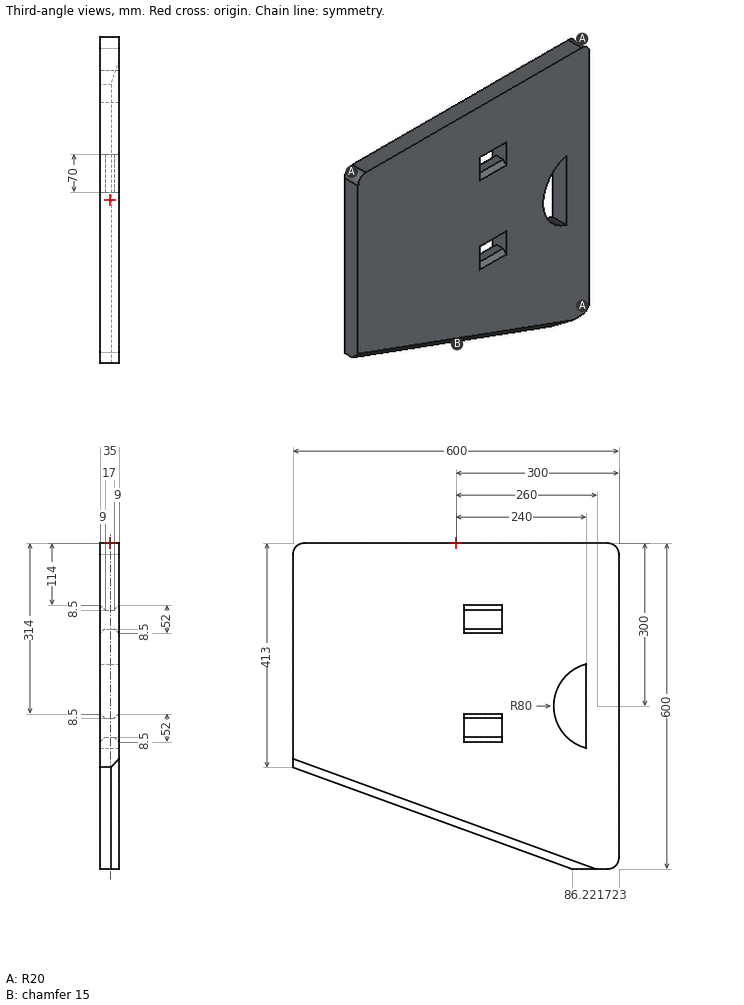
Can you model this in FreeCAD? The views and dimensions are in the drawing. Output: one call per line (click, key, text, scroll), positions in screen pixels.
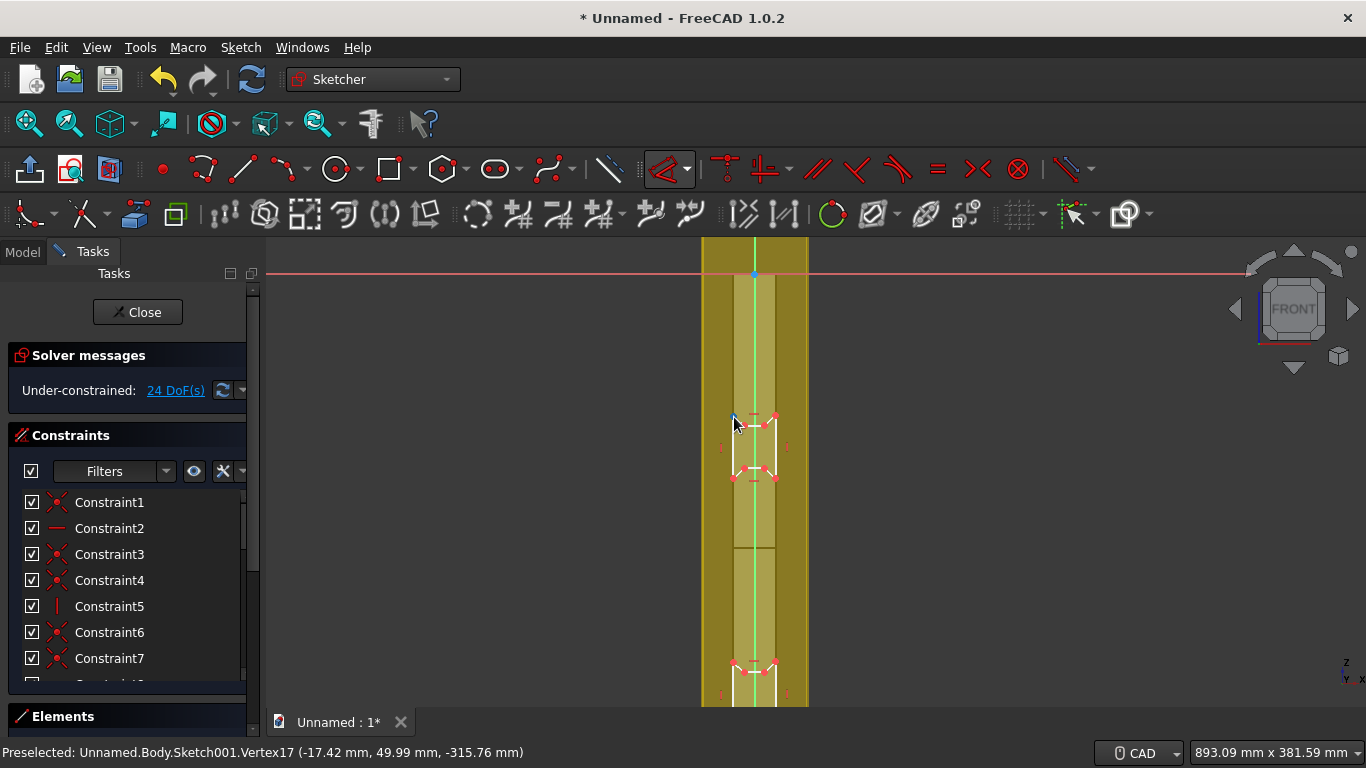
click(733, 416)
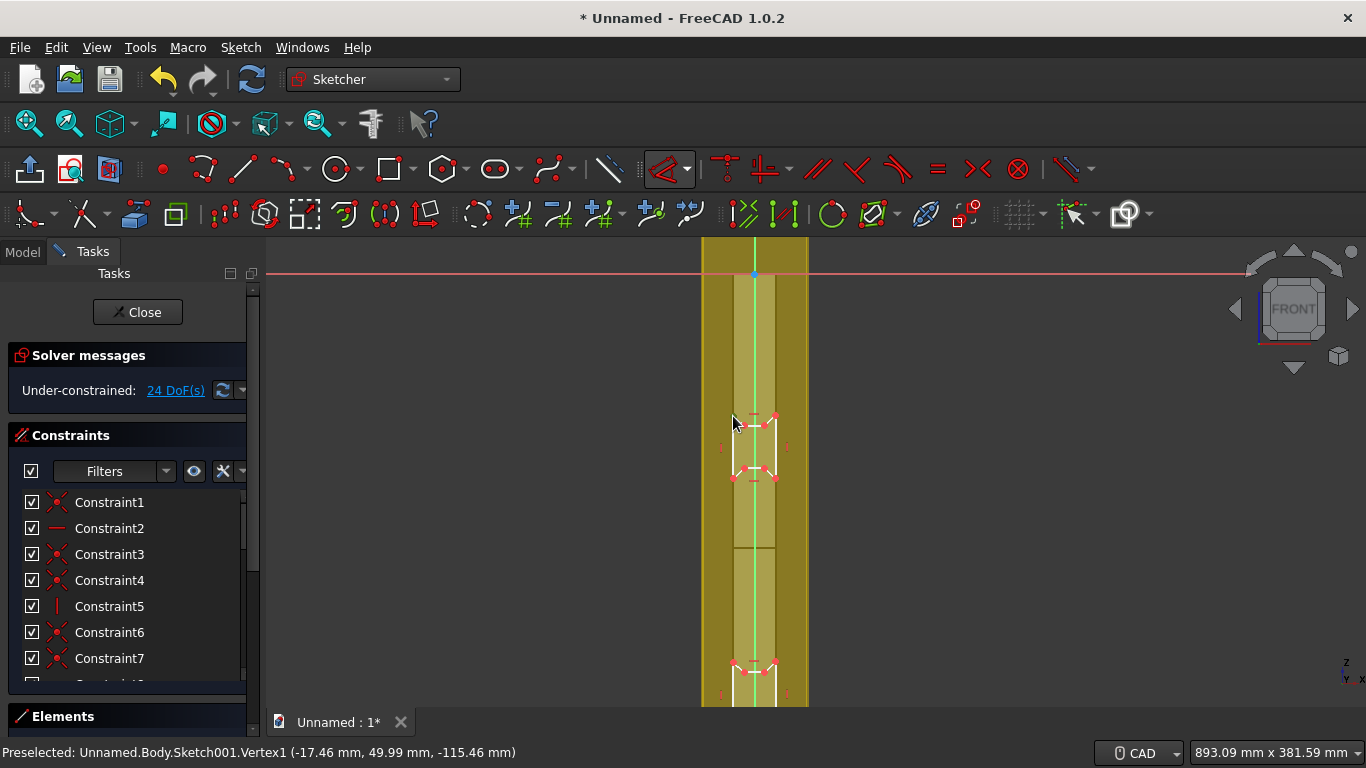
click(776, 415)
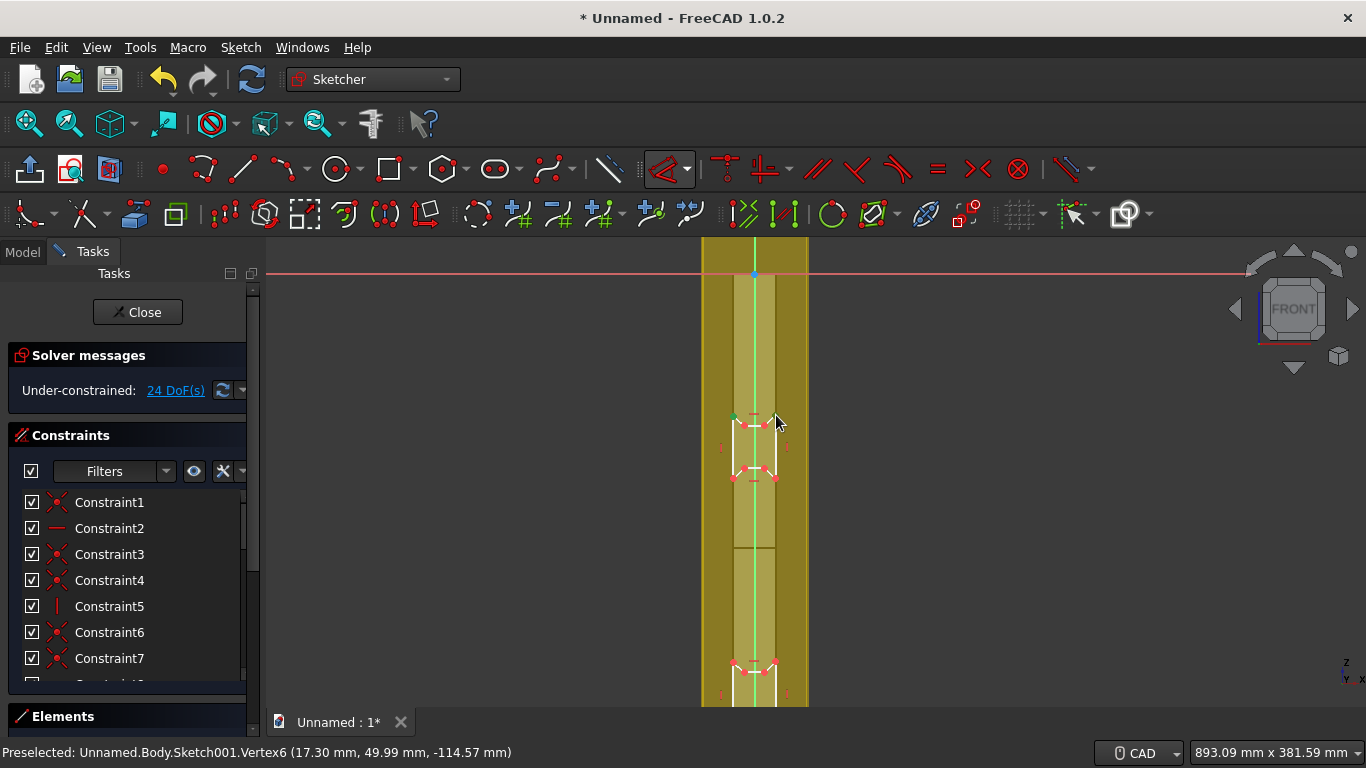
click(755, 620)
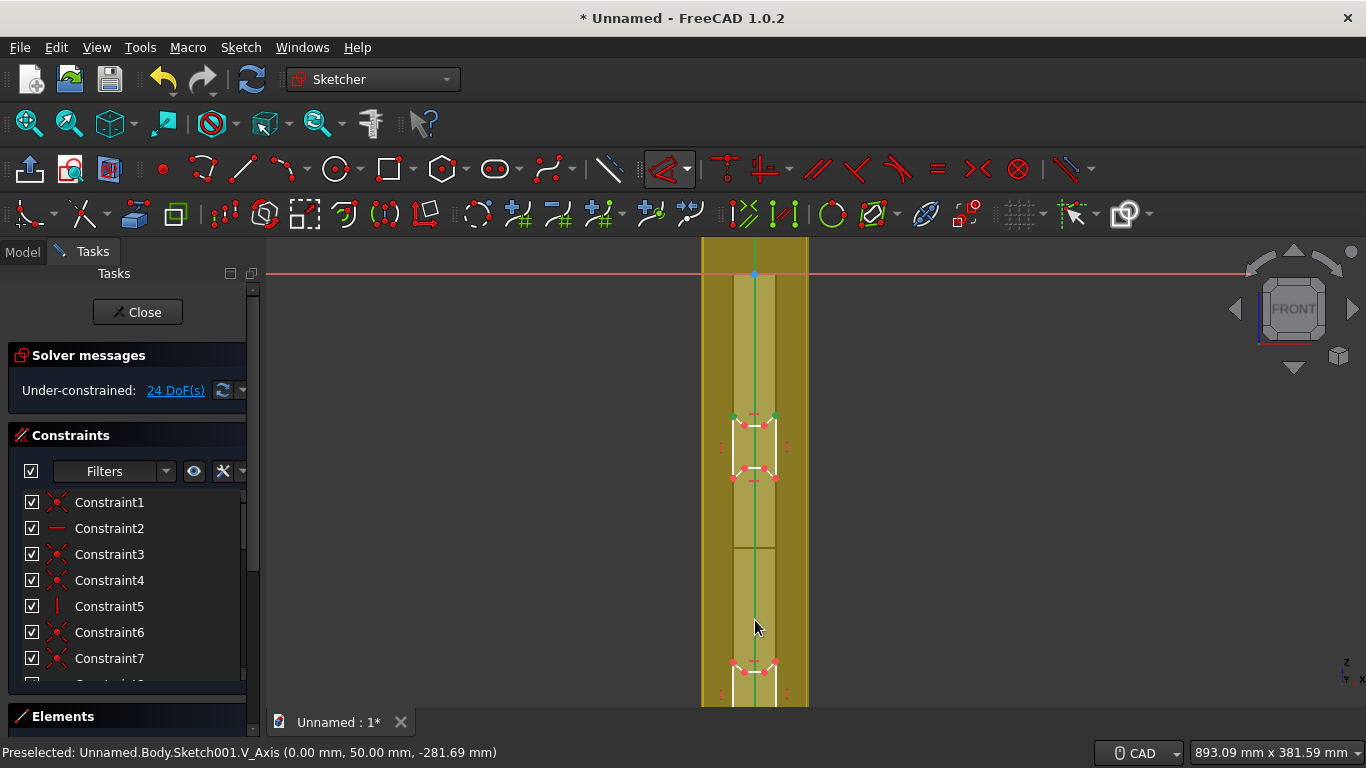
click(978, 170)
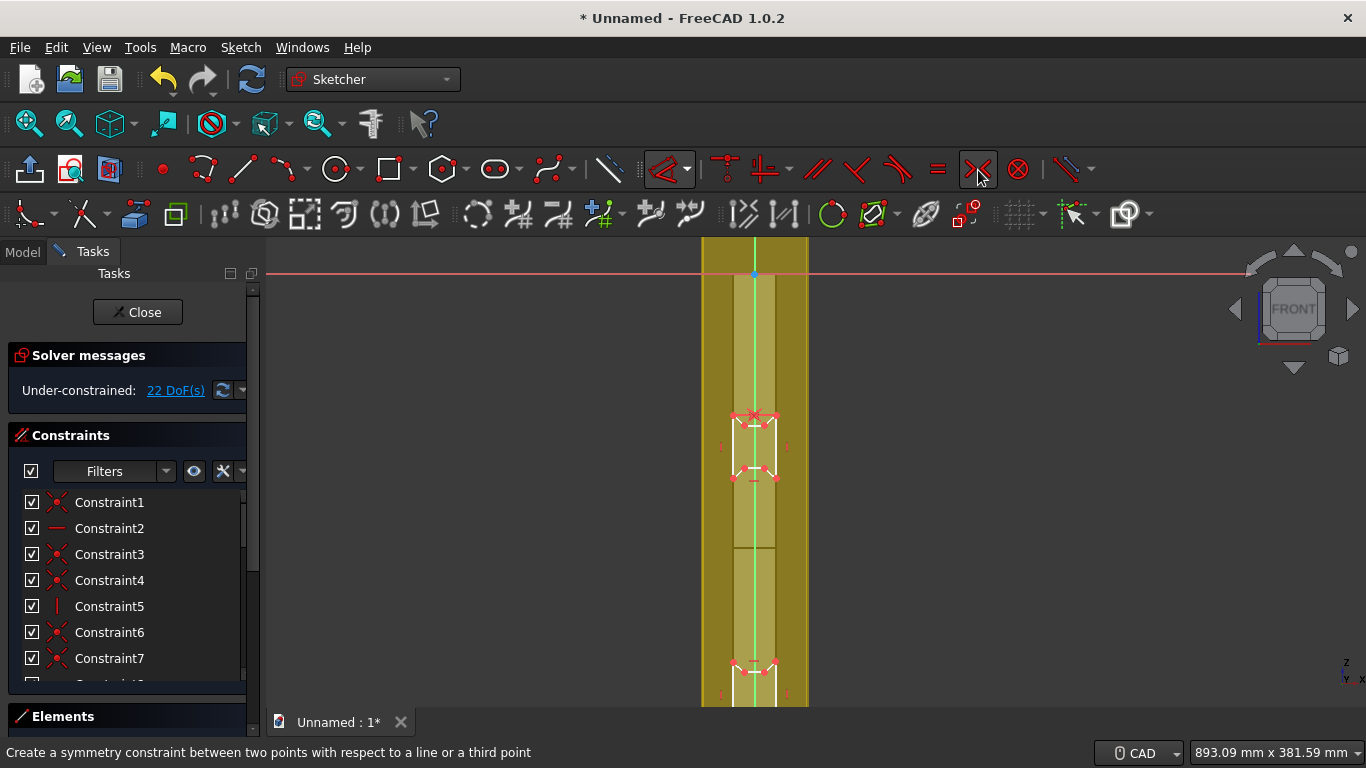
click(733, 663)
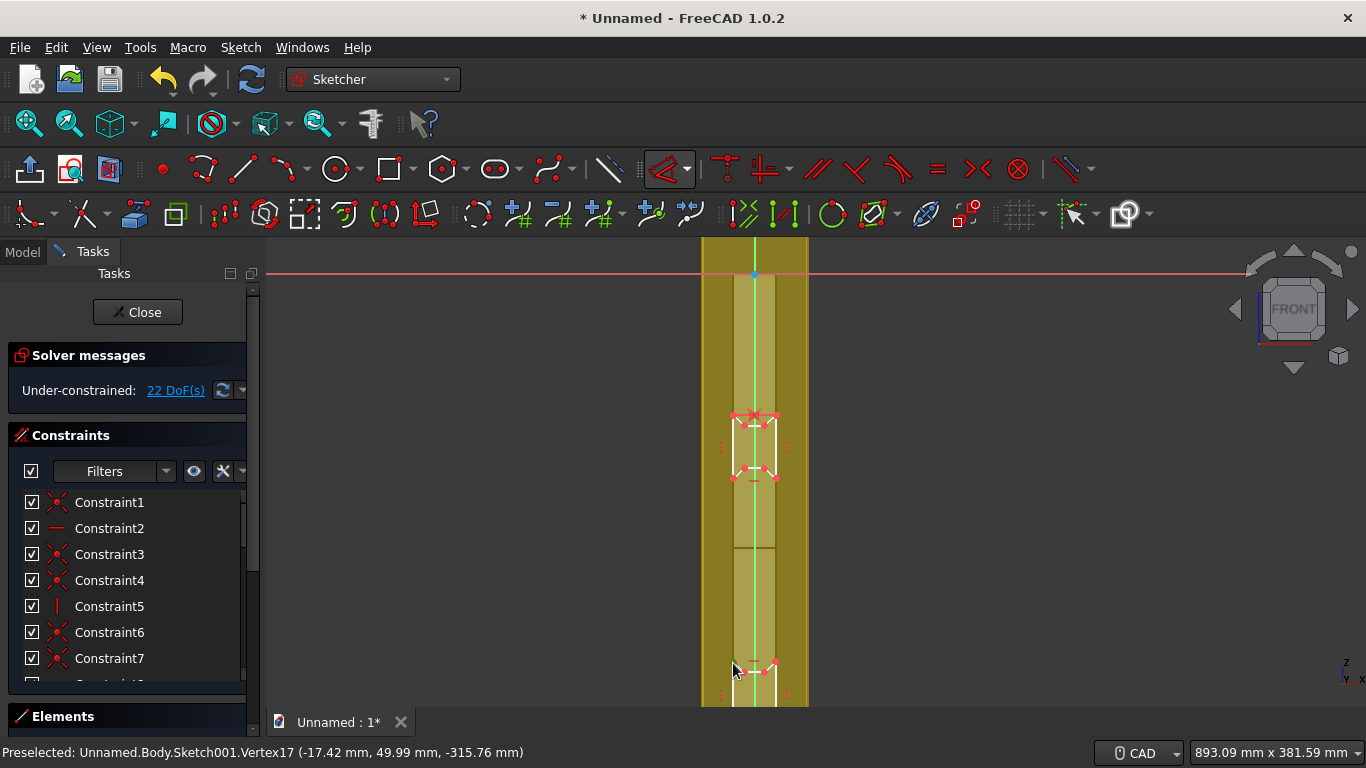
click(776, 661)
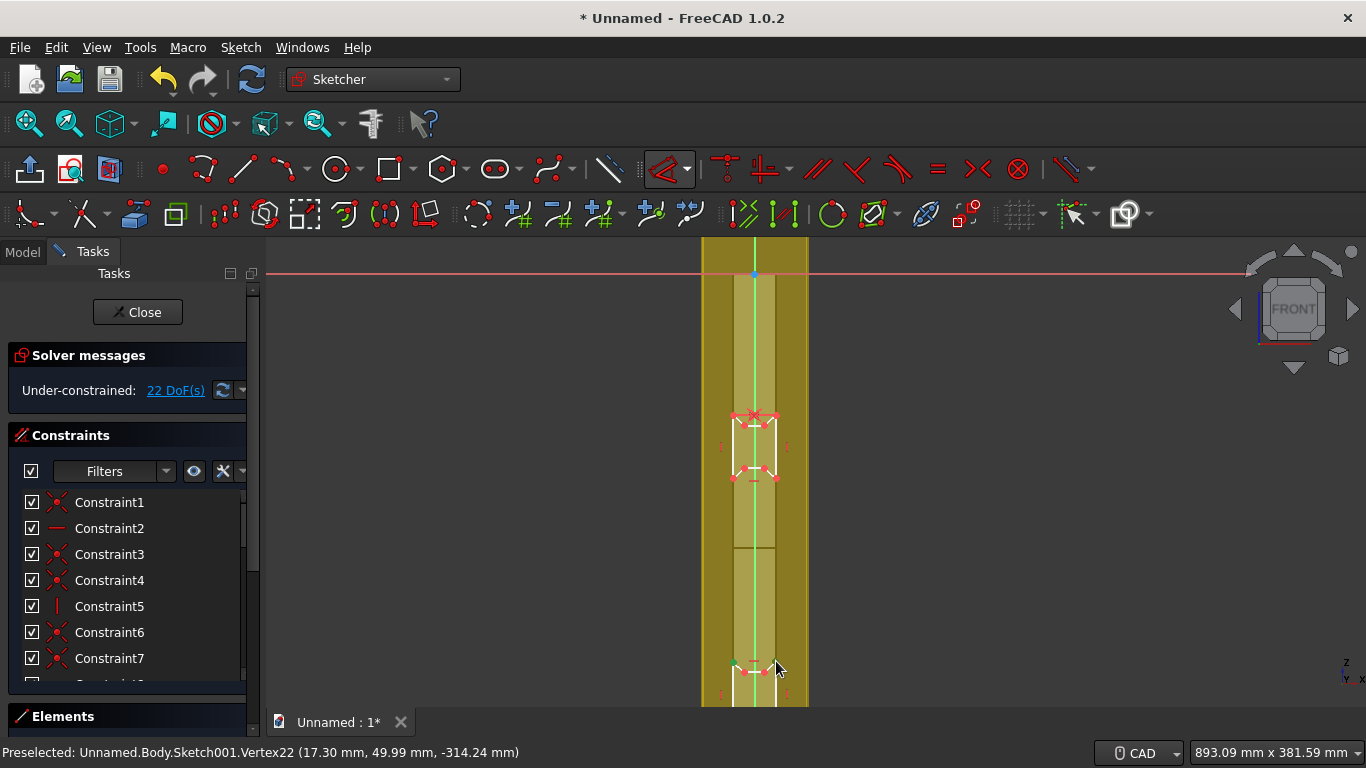
click(755, 620)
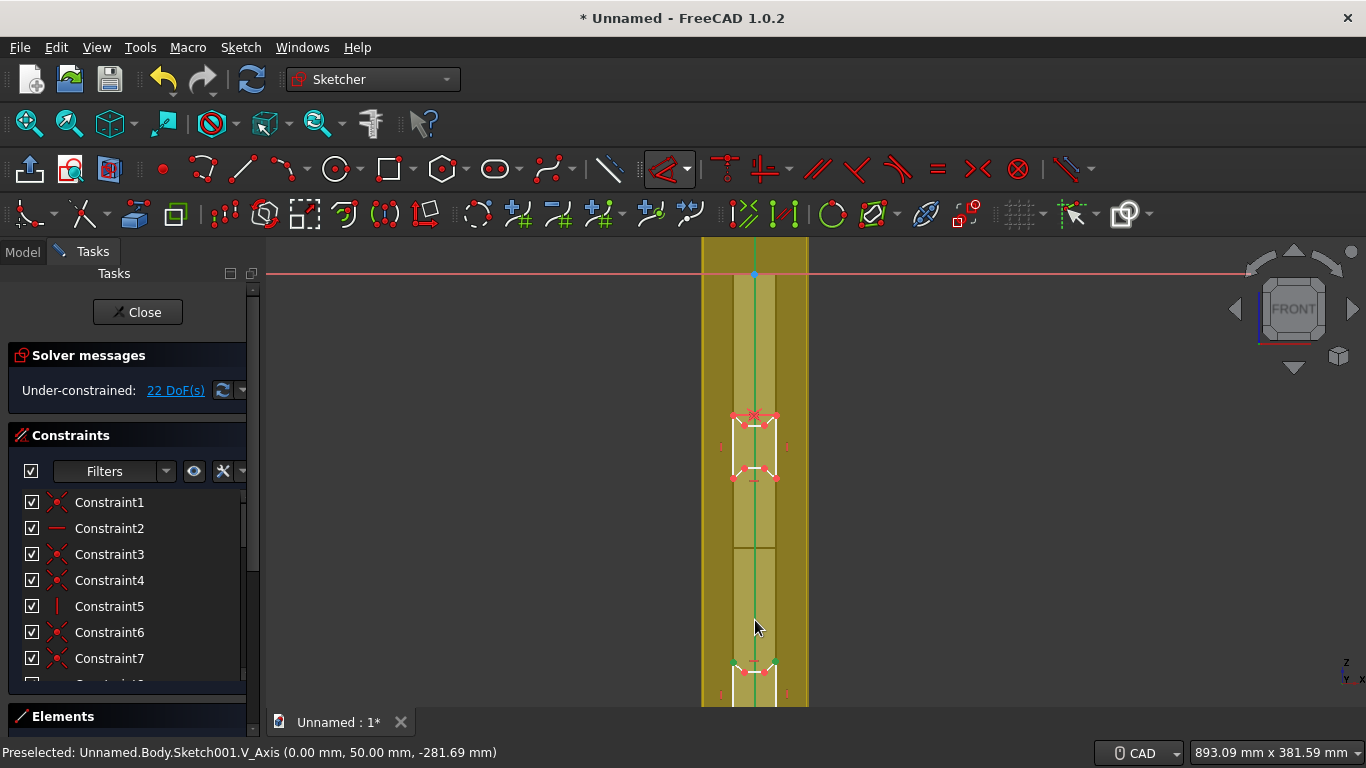
key(s)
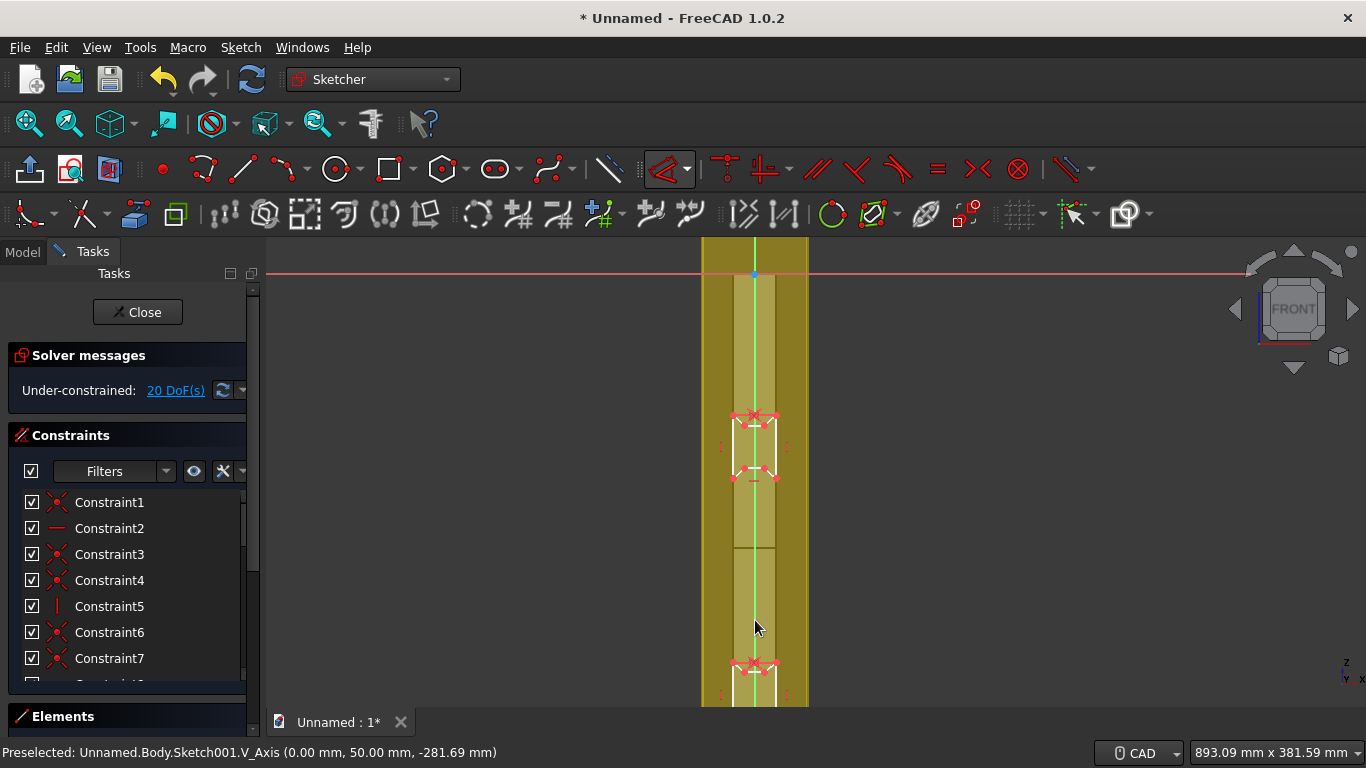
scroll(755, 426, up, 4)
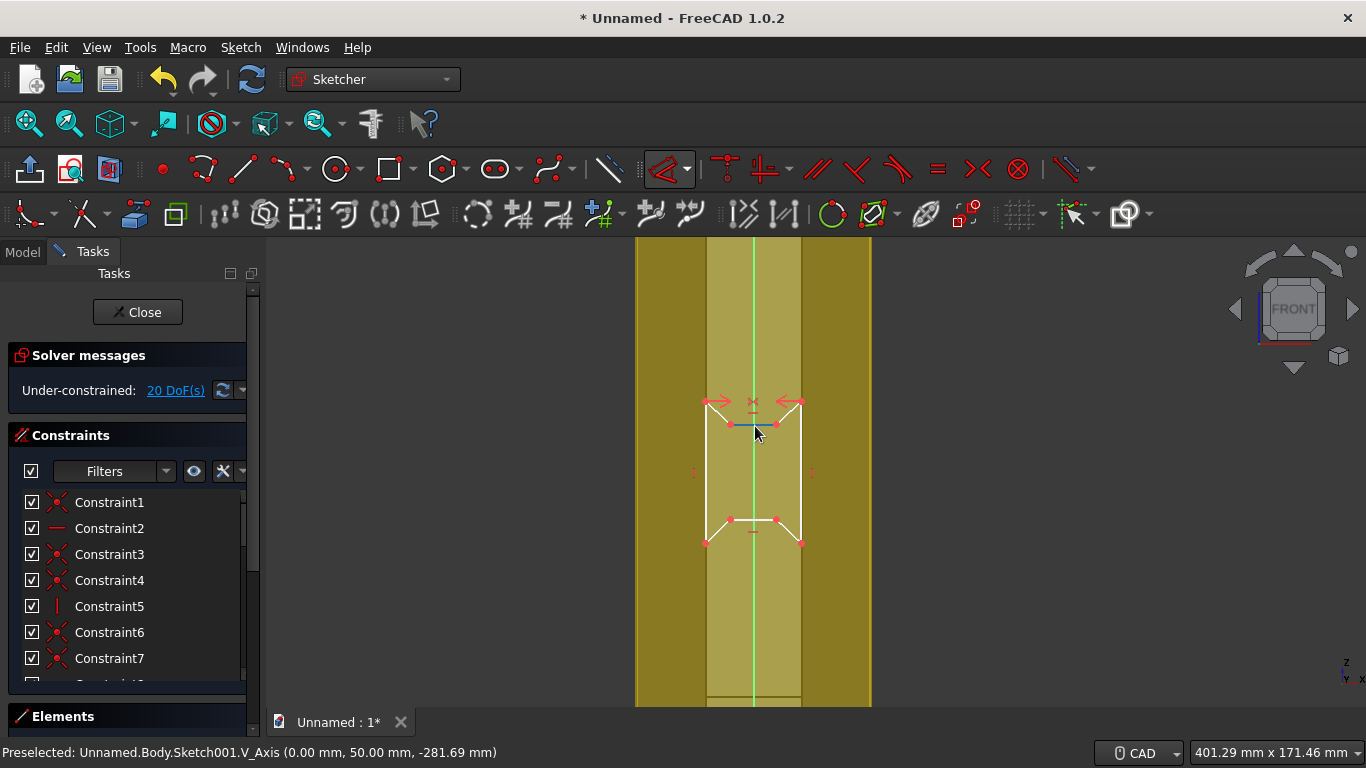
click(753, 425)